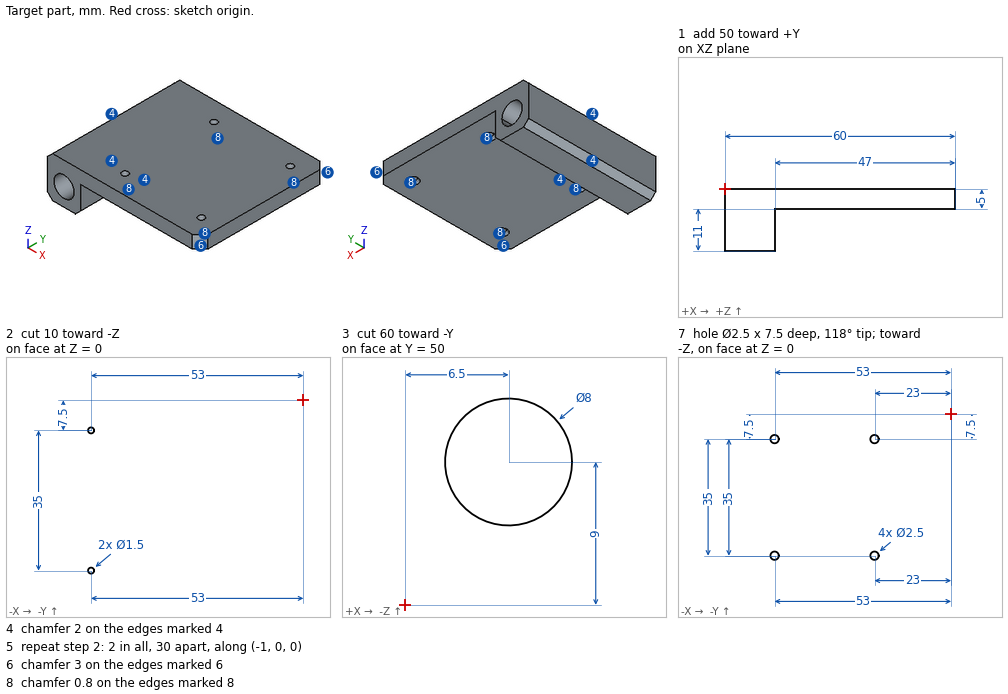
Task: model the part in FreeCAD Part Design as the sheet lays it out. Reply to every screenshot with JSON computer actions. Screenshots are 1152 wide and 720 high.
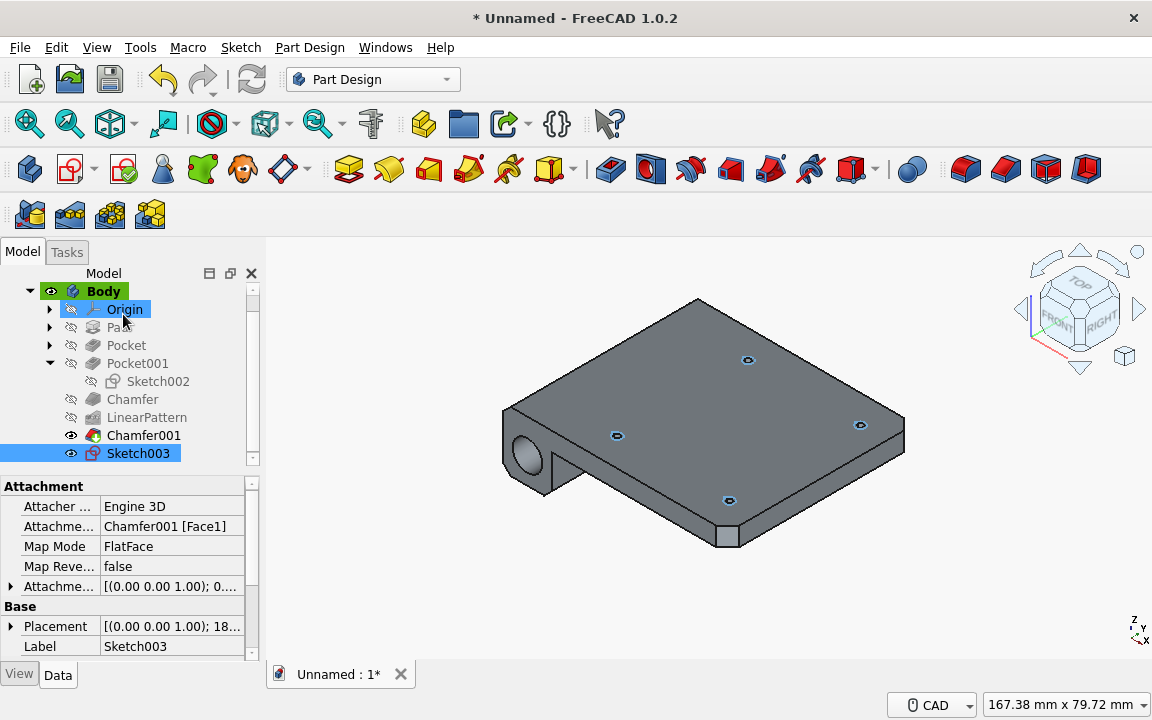
{"action": "left_click", "coordinate": [652, 170]}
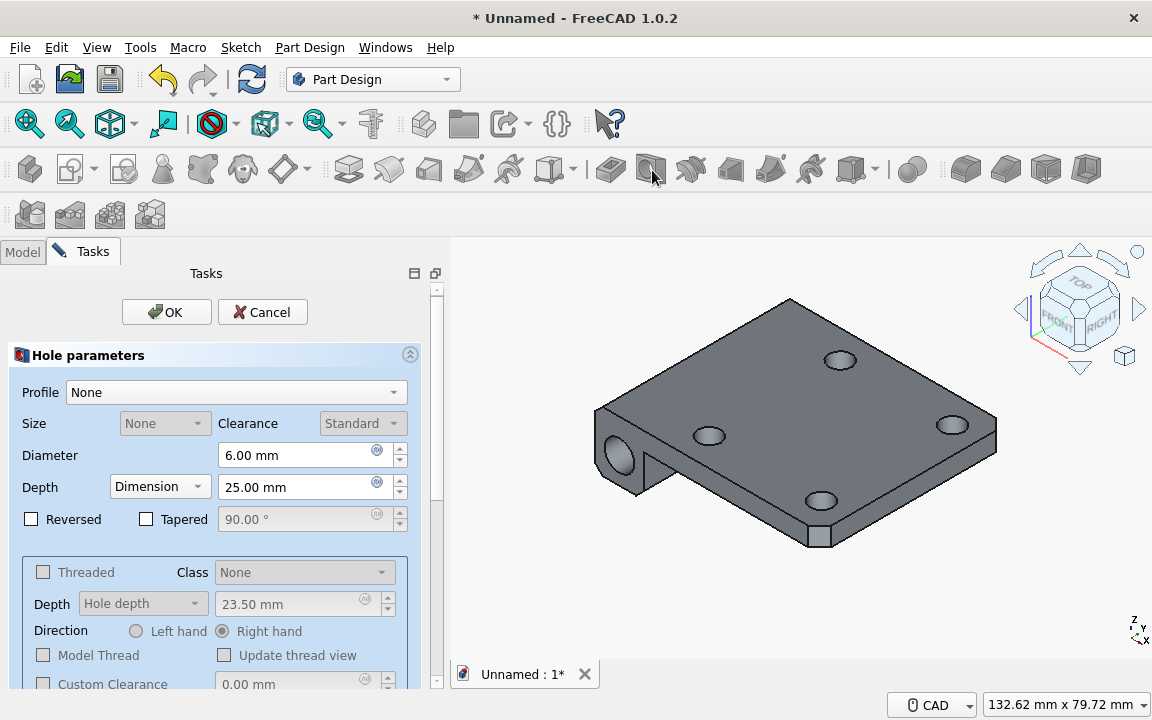
{"action": "triple_click", "coordinate": [305, 455]}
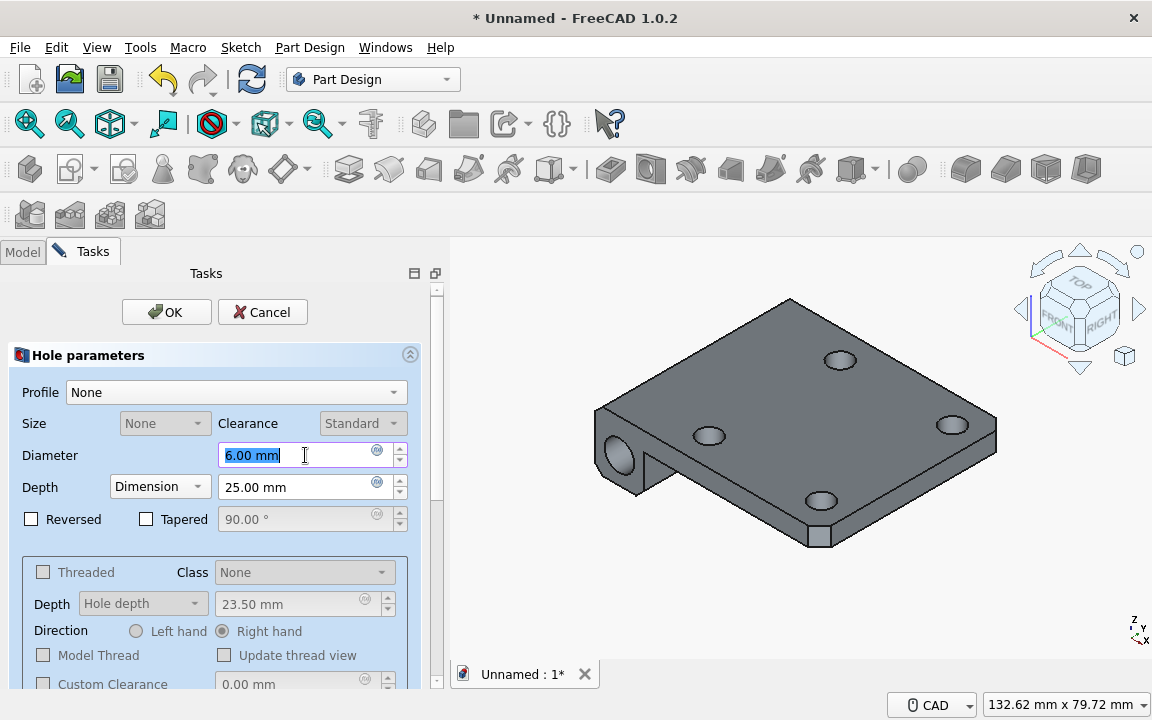
{"action": "type", "text": "2.5"}
{"action": "key", "text": "Tab"}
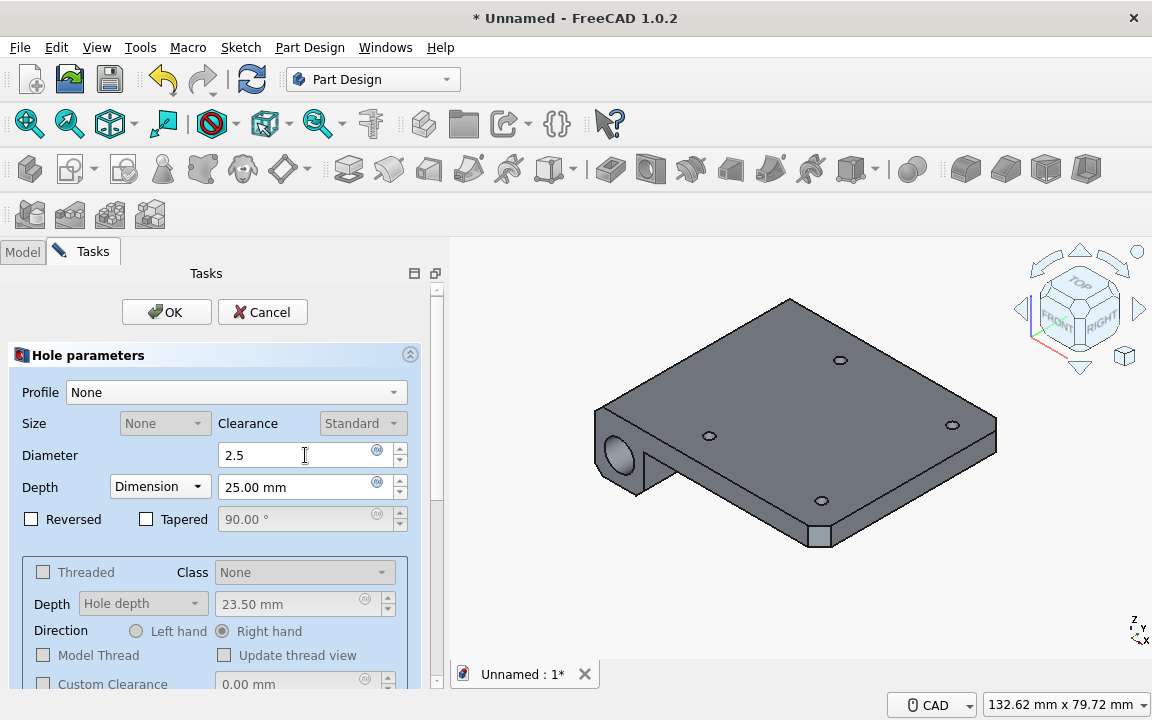
{"action": "triple_click", "coordinate": [305, 487]}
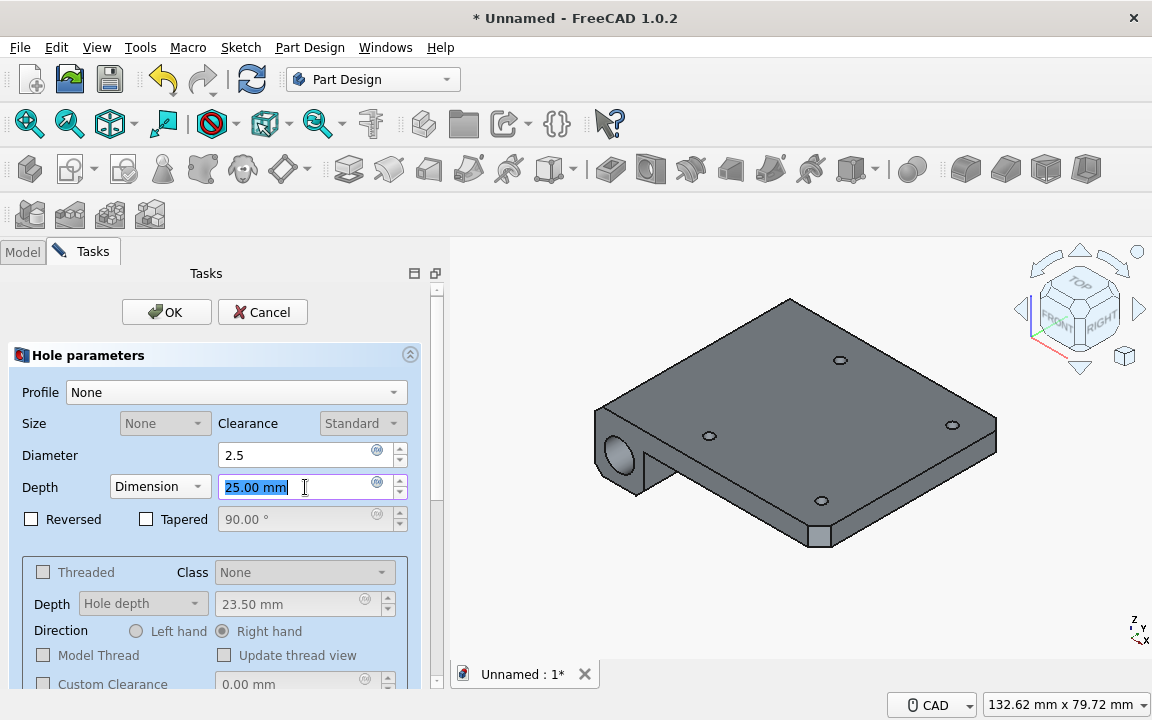
{"action": "type", "text": "7.5"}
{"action": "key", "text": "Tab"}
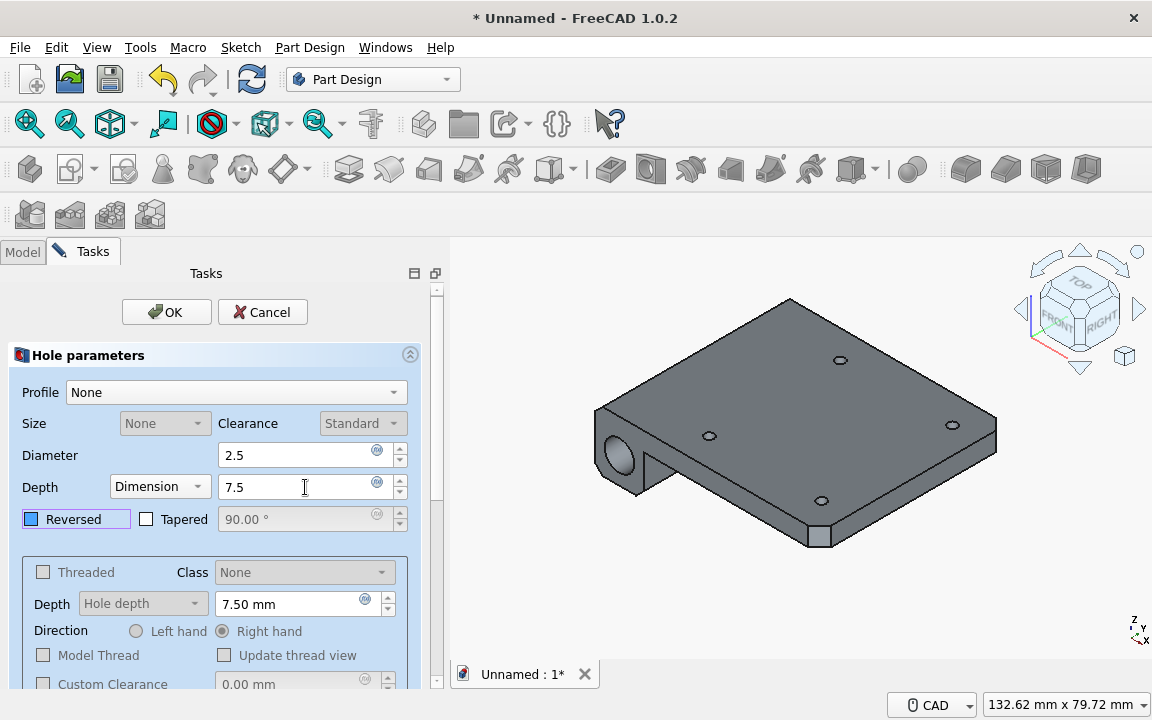
{"action": "left_click", "coordinate": [167, 312]}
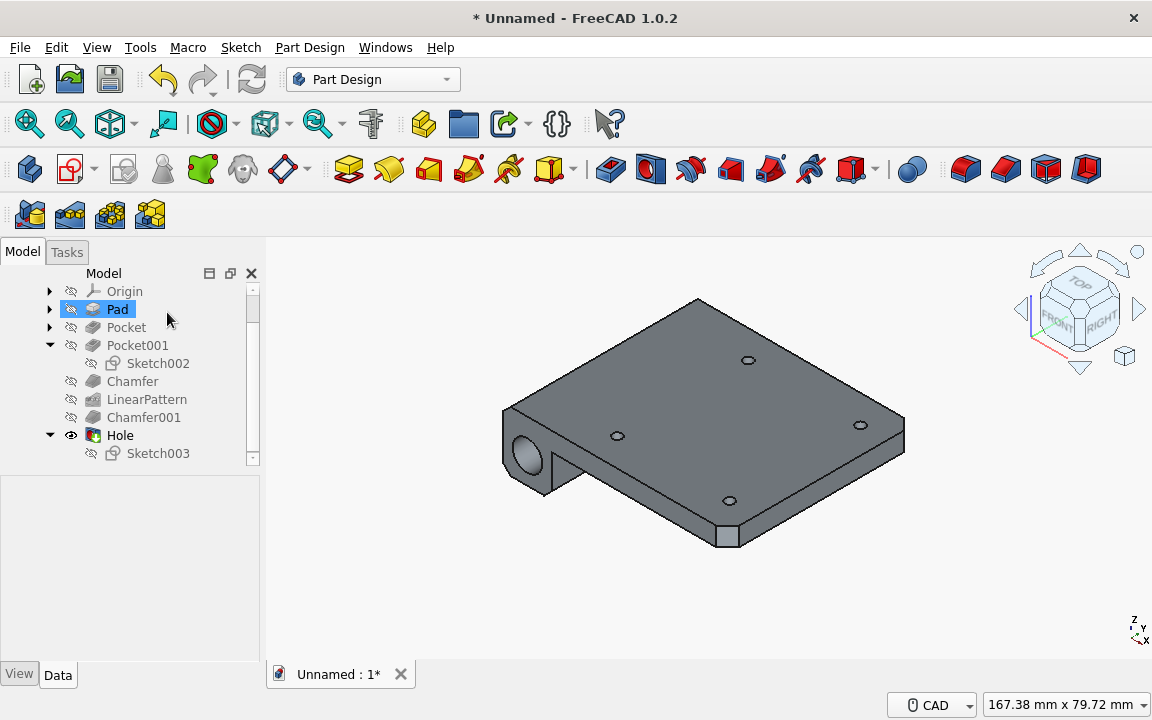
{"action": "key", "text": "2"}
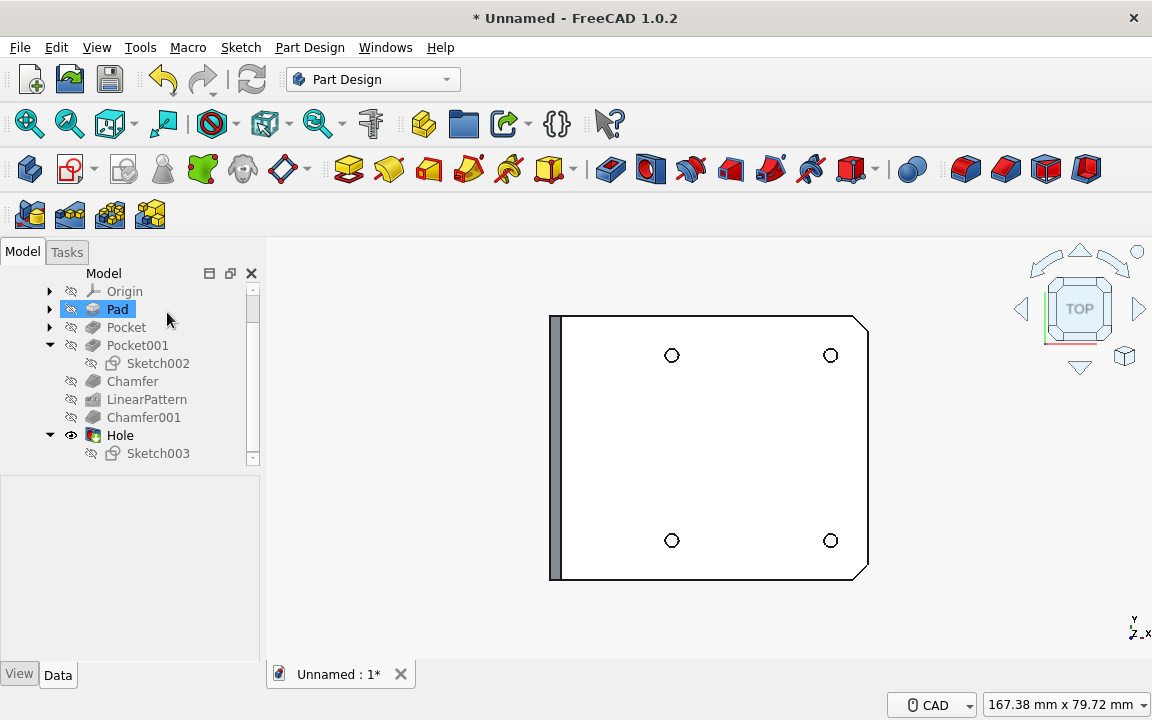
{"action": "key", "text": "0"}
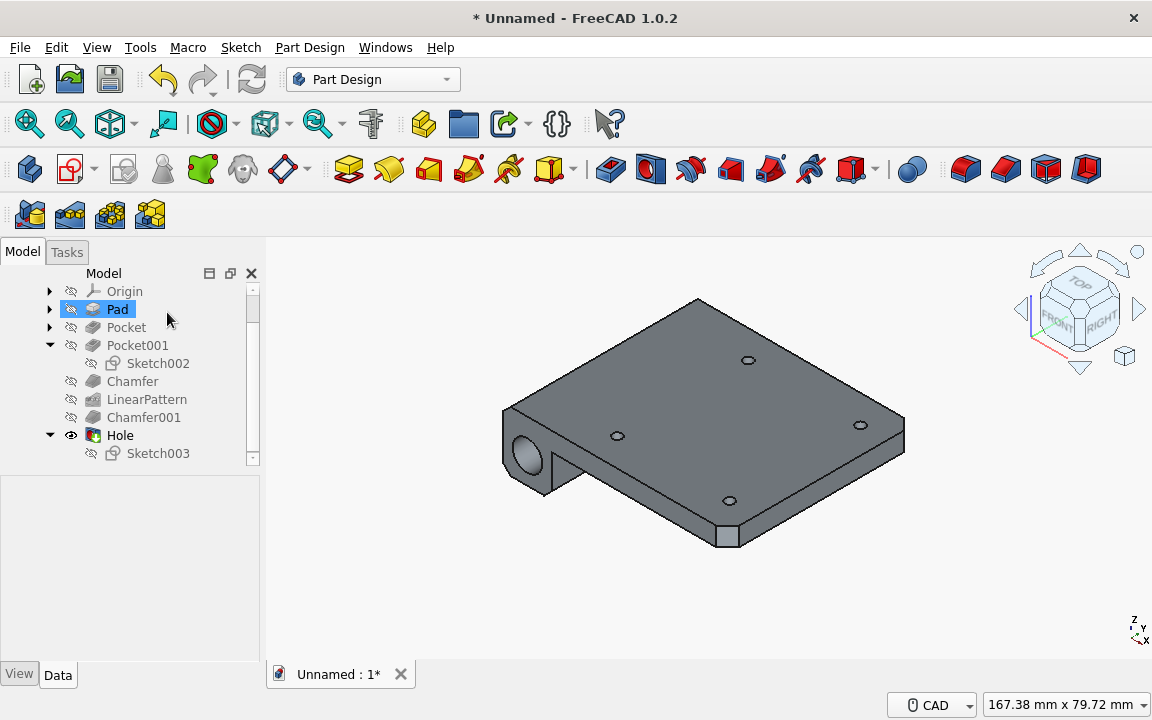
{"action": "key", "text": "1"}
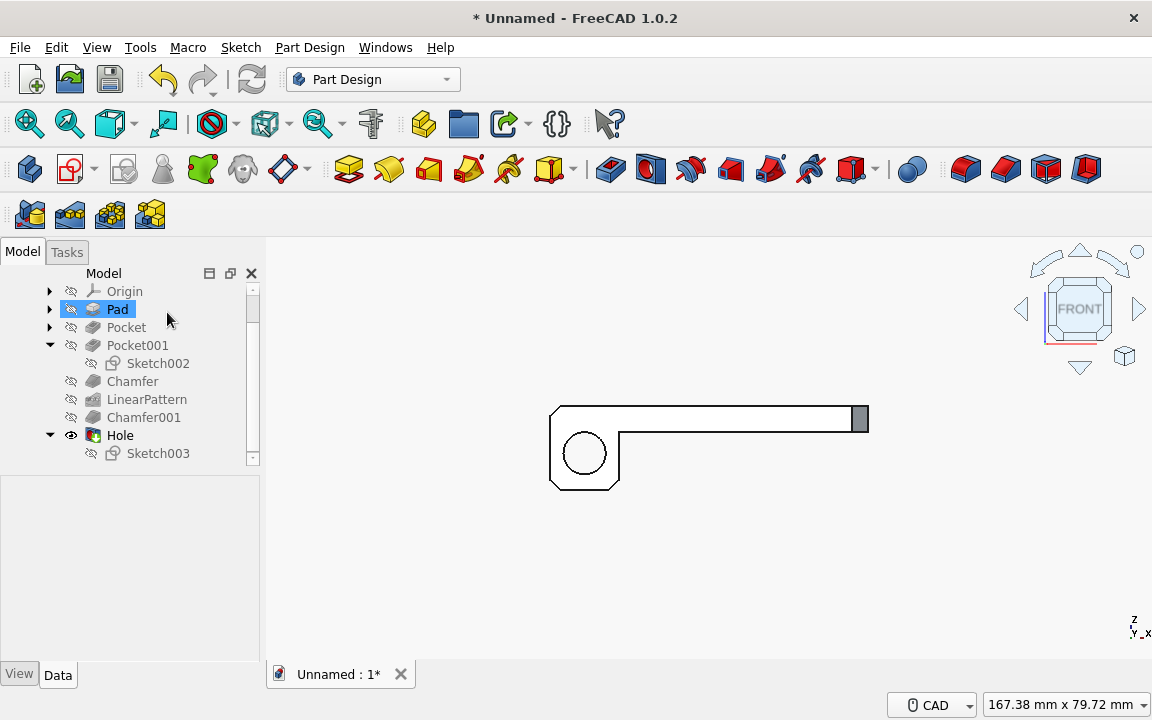
{"action": "left_click", "coordinate": [30, 124]}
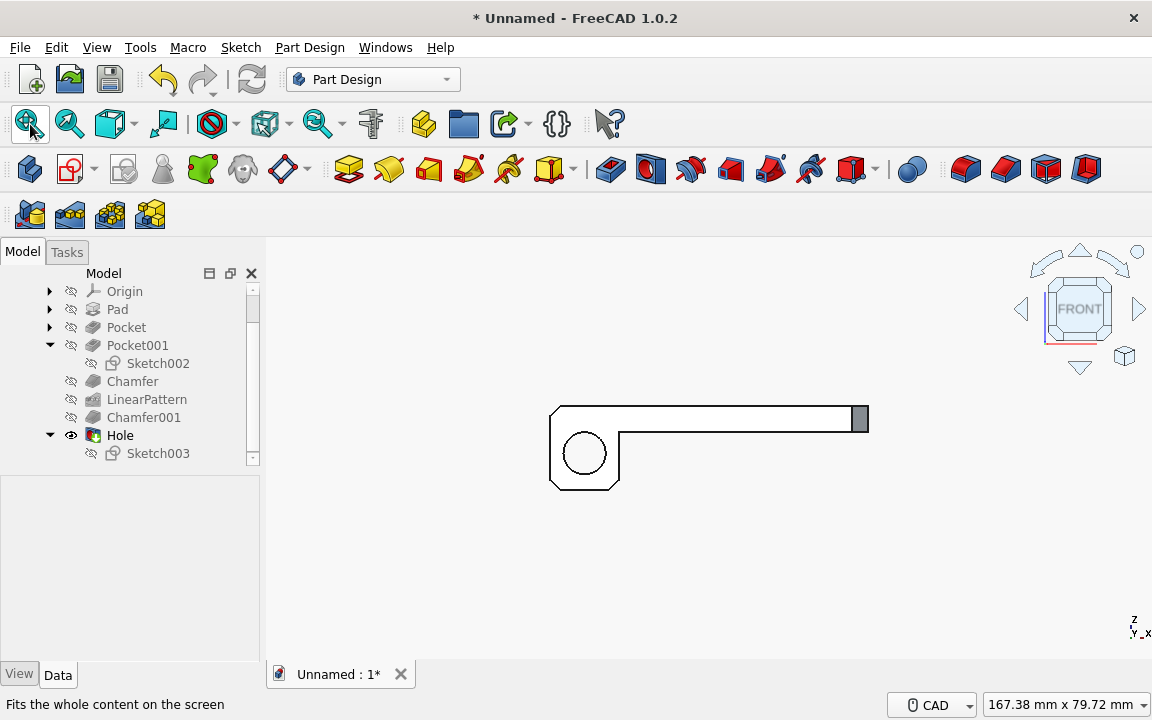
{"action": "key", "text": "3"}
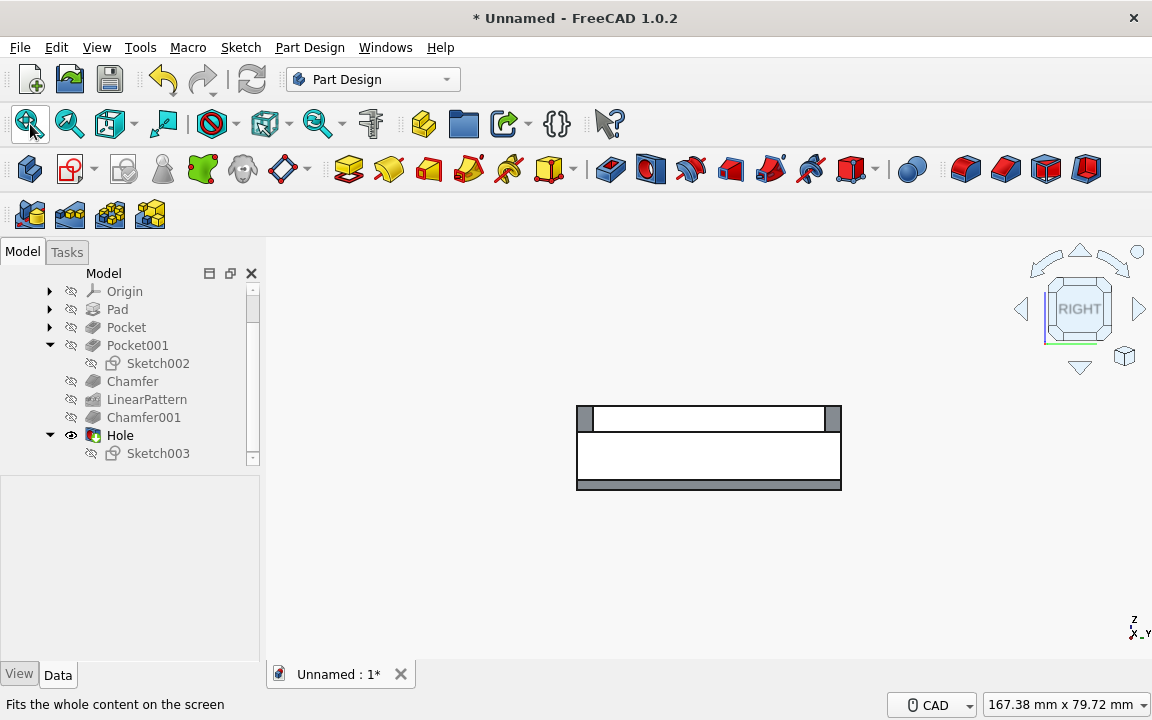
{"action": "left_click", "coordinate": [30, 124]}